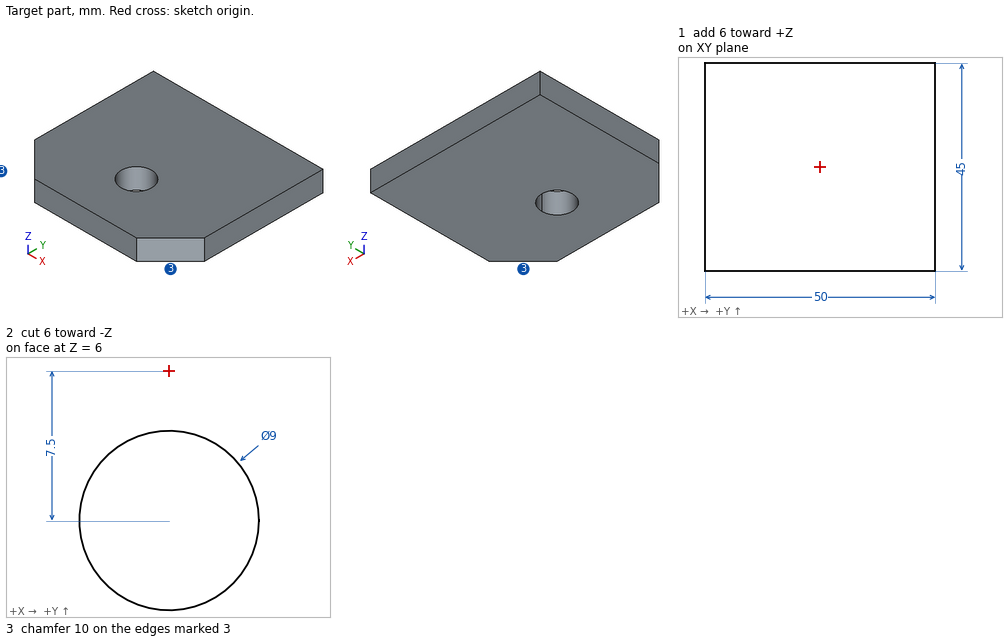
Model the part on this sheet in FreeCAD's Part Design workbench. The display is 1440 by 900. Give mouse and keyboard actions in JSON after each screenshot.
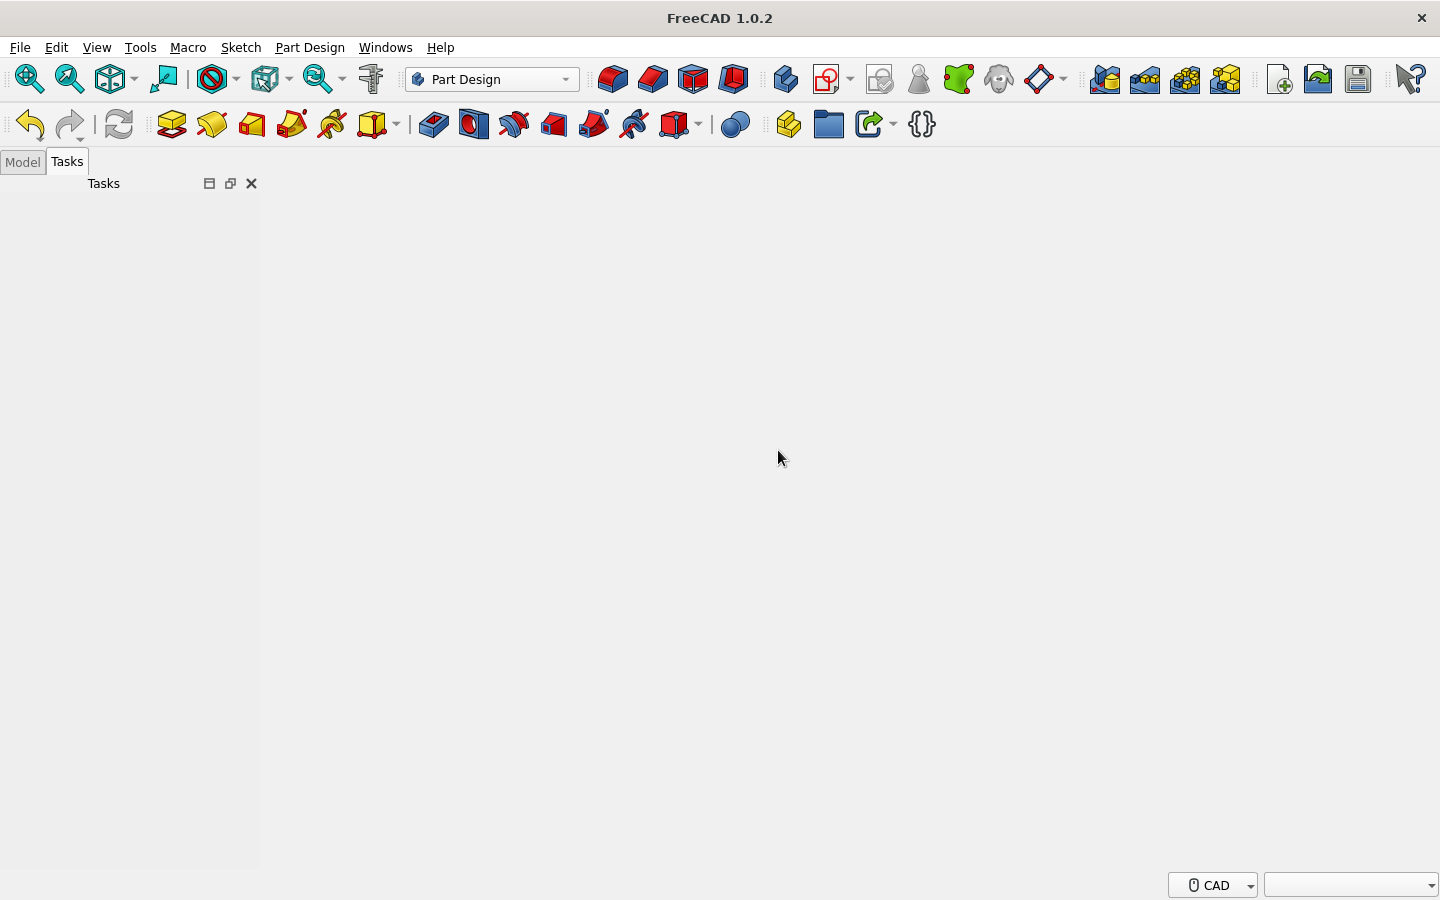
{"action": "key", "text": "ctrl+n"}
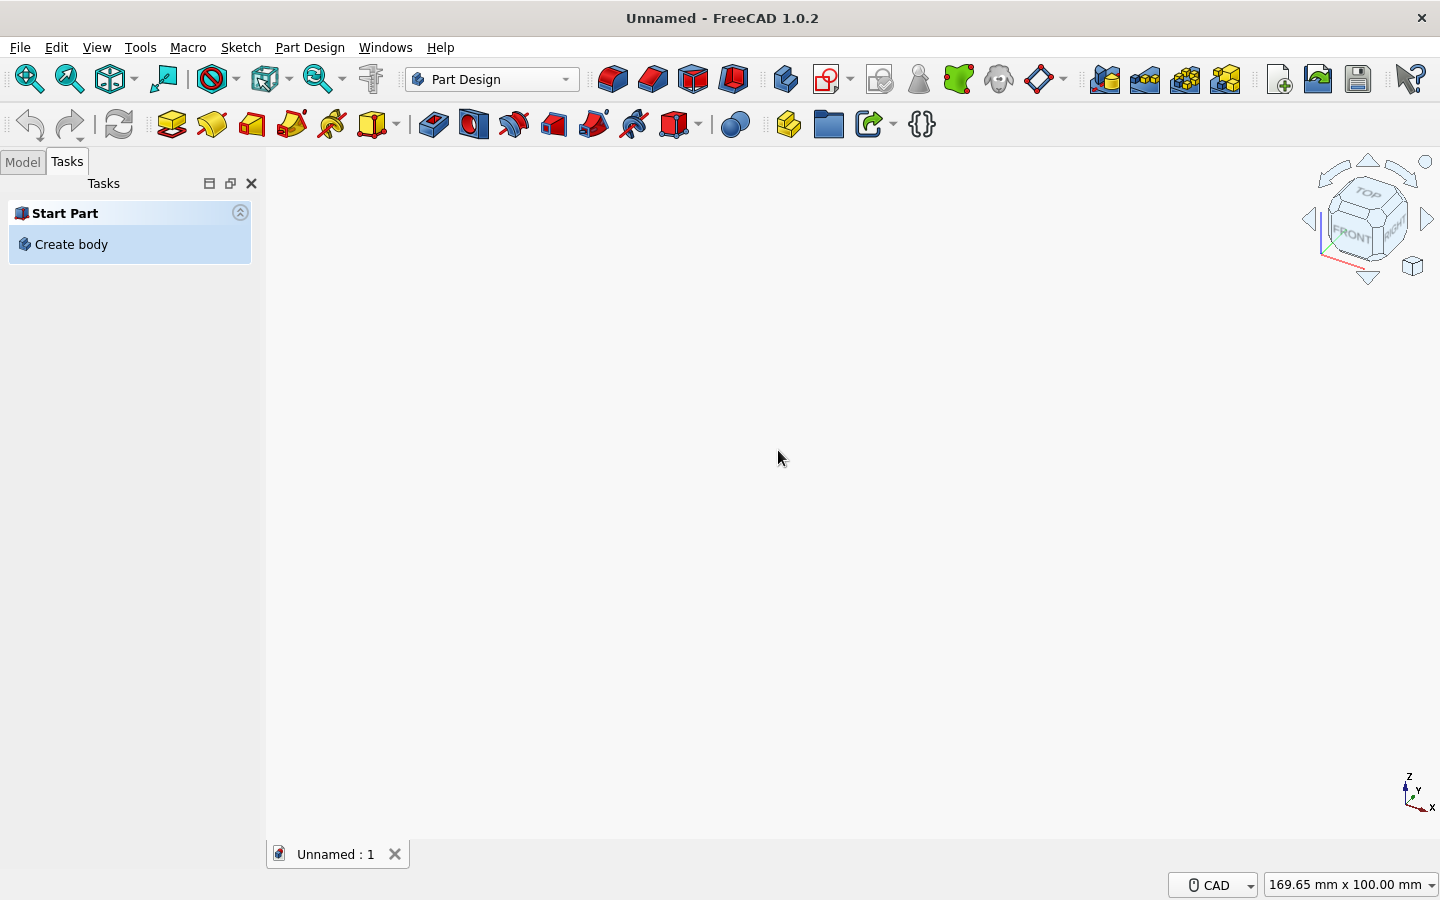
{"action": "left_click", "coordinate": [826, 80]}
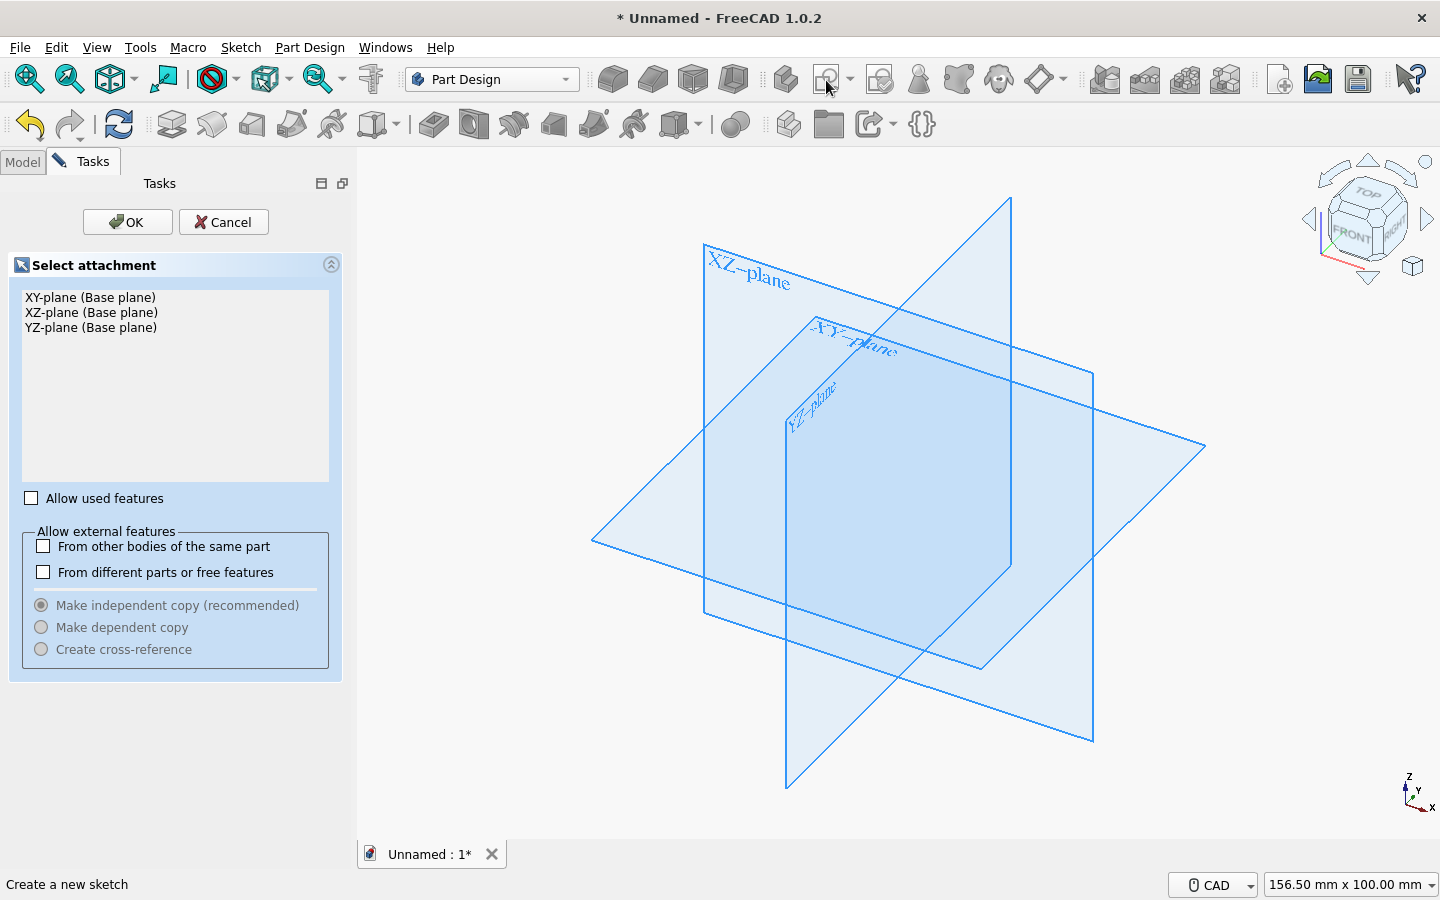
{"action": "left_click", "coordinate": [82, 298]}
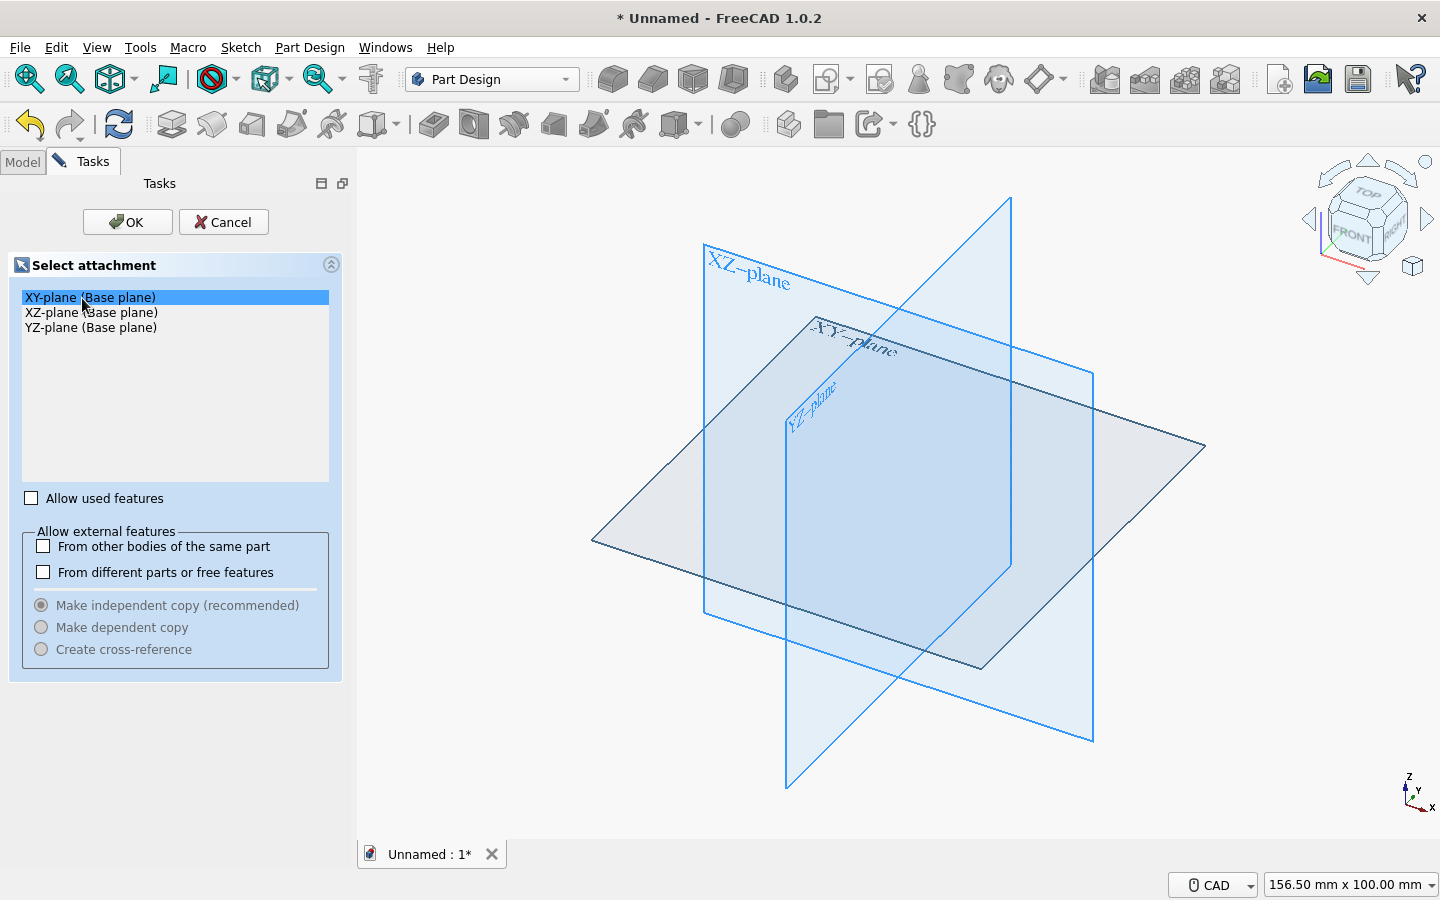
{"action": "left_click", "coordinate": [128, 222]}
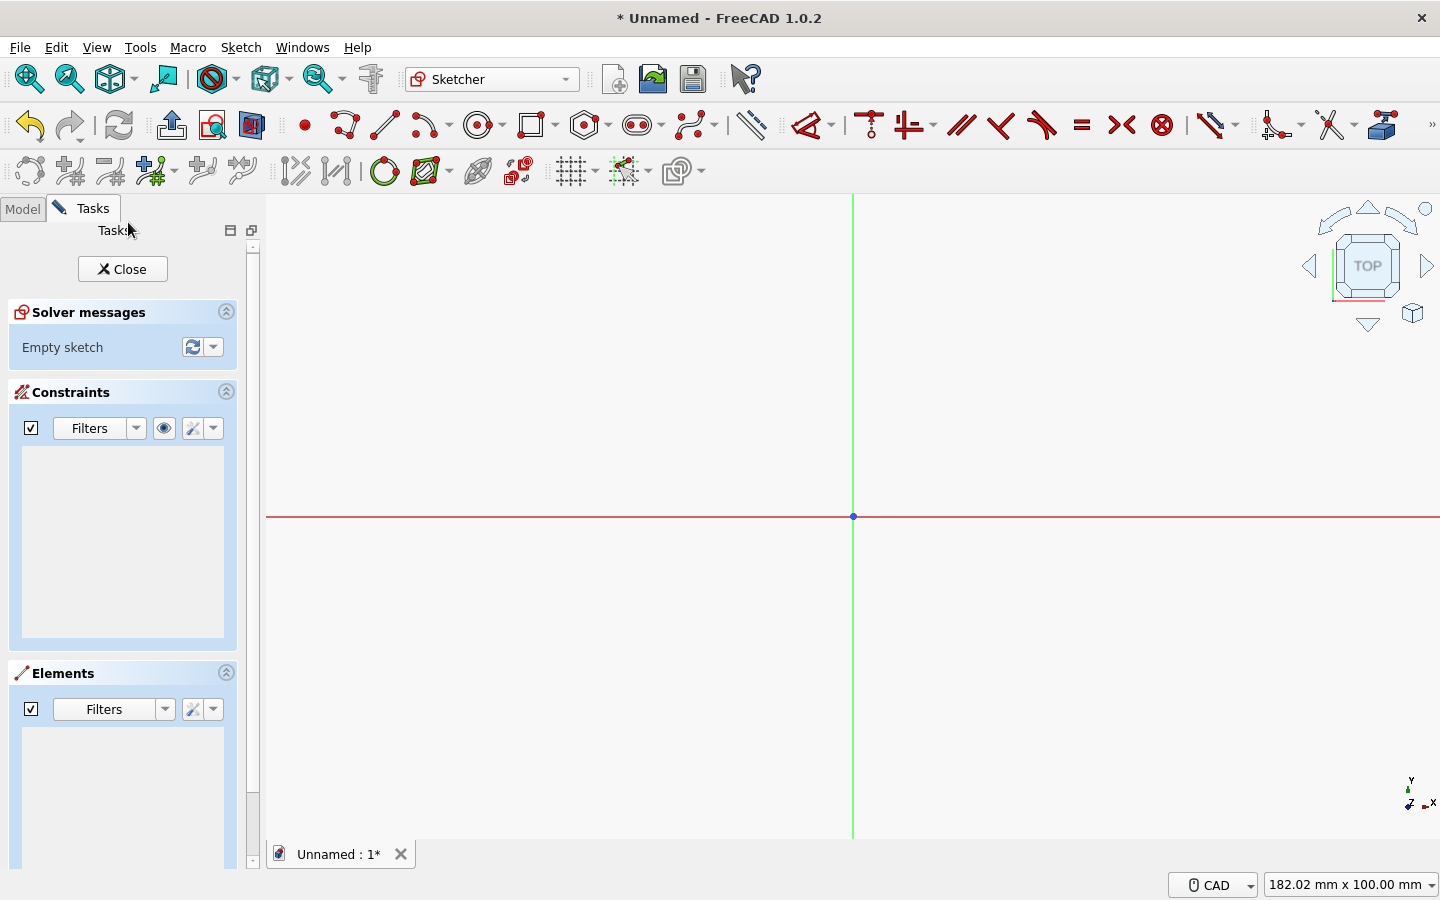
{"action": "scroll", "coordinate": [992, 517], "scroll_direction": "up", "scroll_amount": 2}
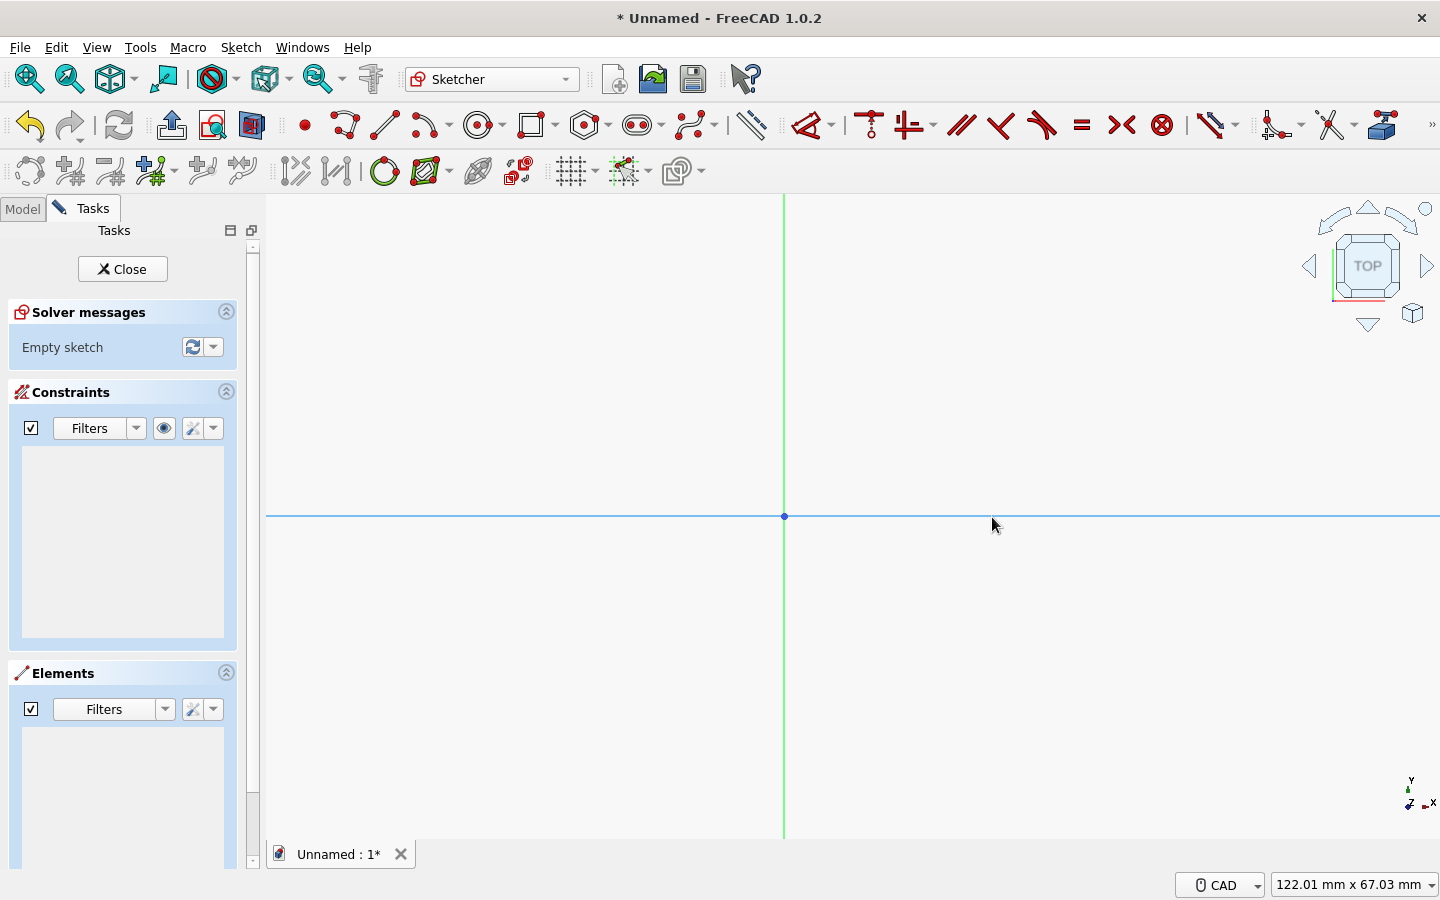
{"action": "key", "text": "g v"}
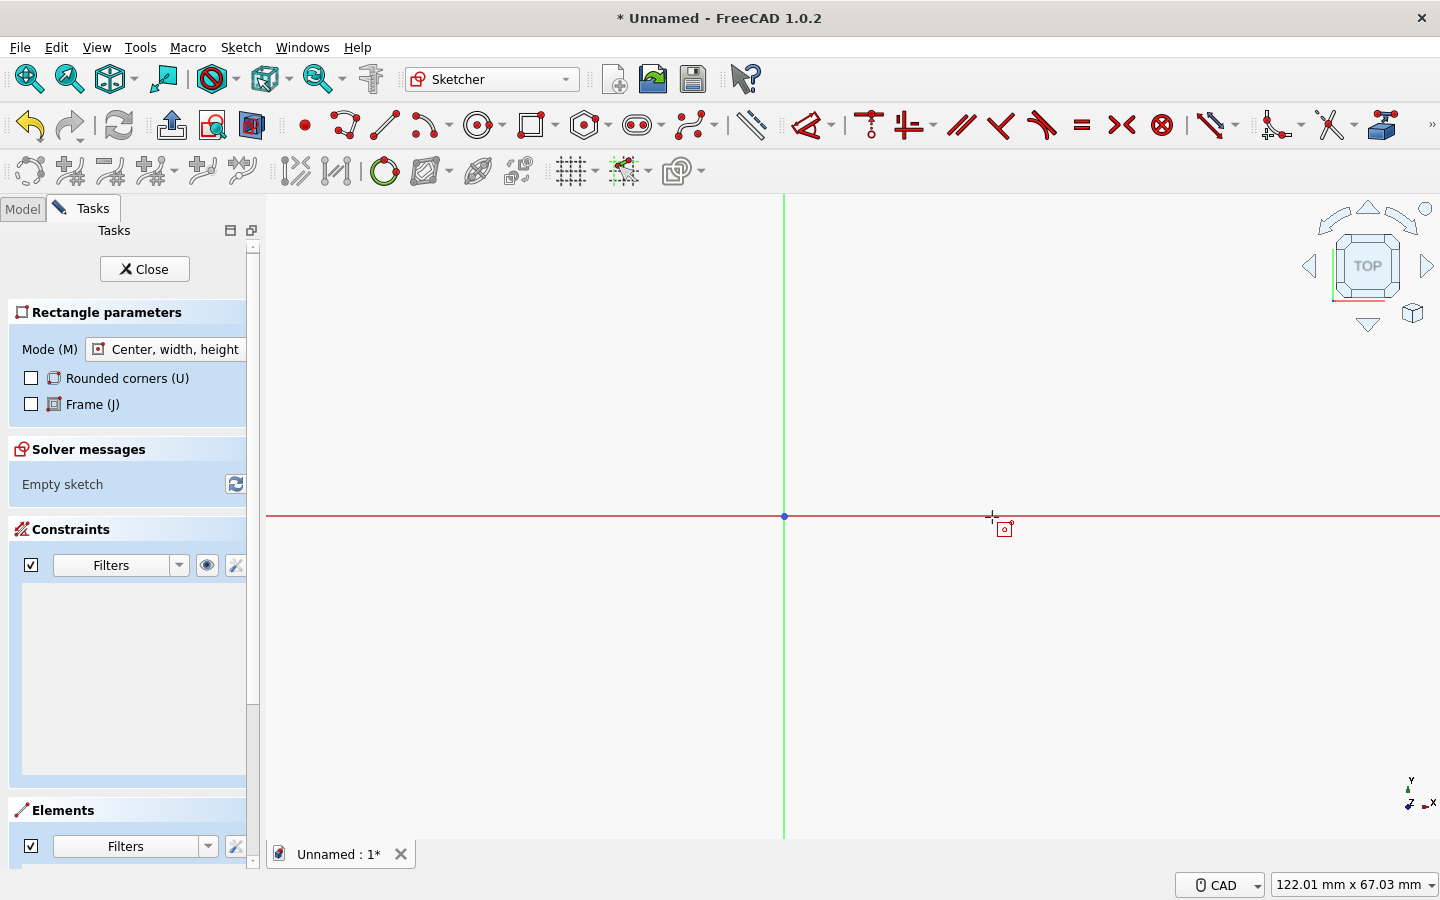
{"action": "left_click", "coordinate": [784, 516]}
{"action": "mouse_move", "coordinate": [1025, 300]}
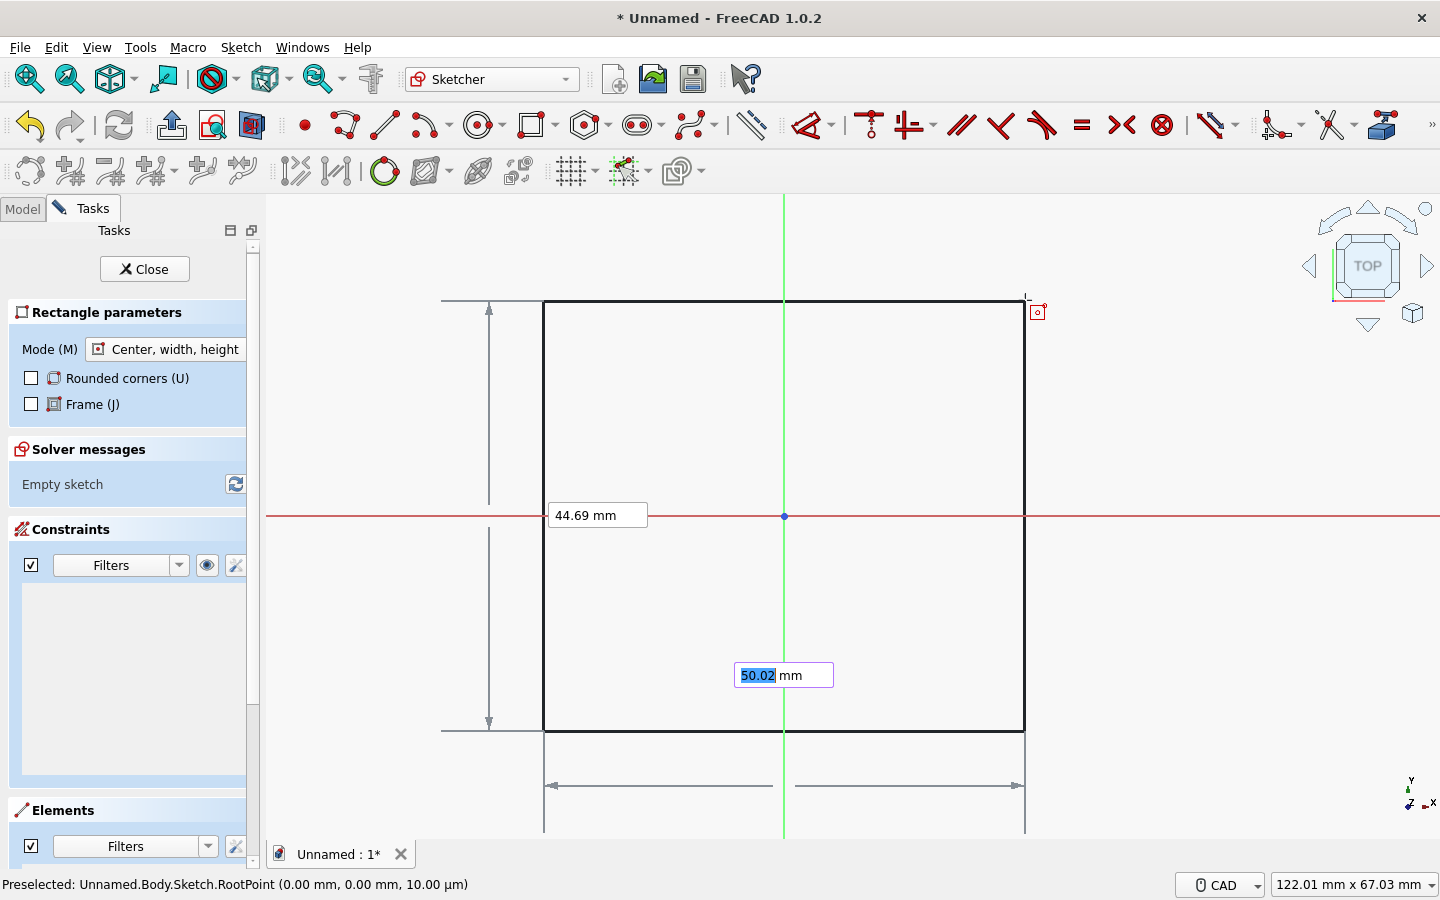
{"action": "type", "text": "50"}
{"action": "key", "text": "Tab"}
{"action": "type", "text": "45"}
{"action": "key", "text": "Return"}
{"action": "key", "text": "Escape"}